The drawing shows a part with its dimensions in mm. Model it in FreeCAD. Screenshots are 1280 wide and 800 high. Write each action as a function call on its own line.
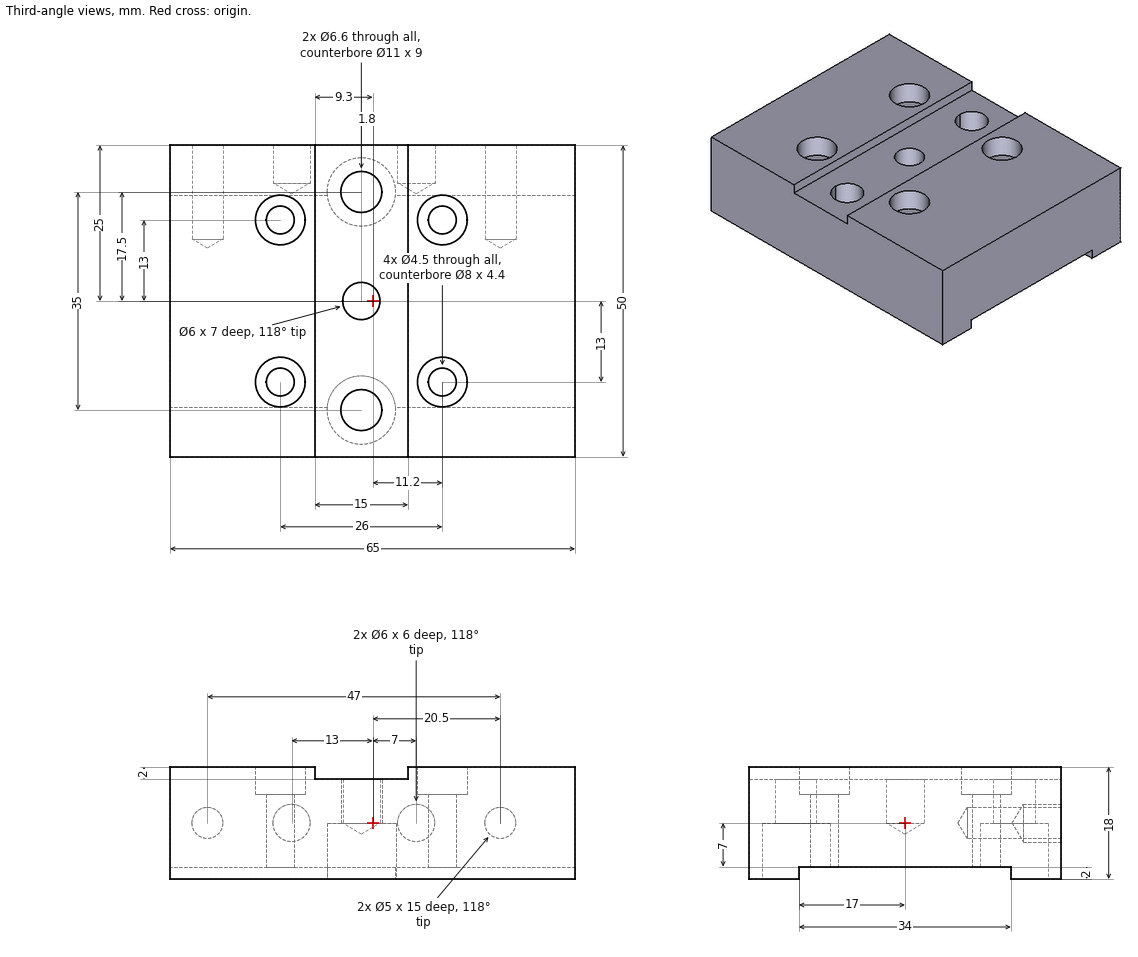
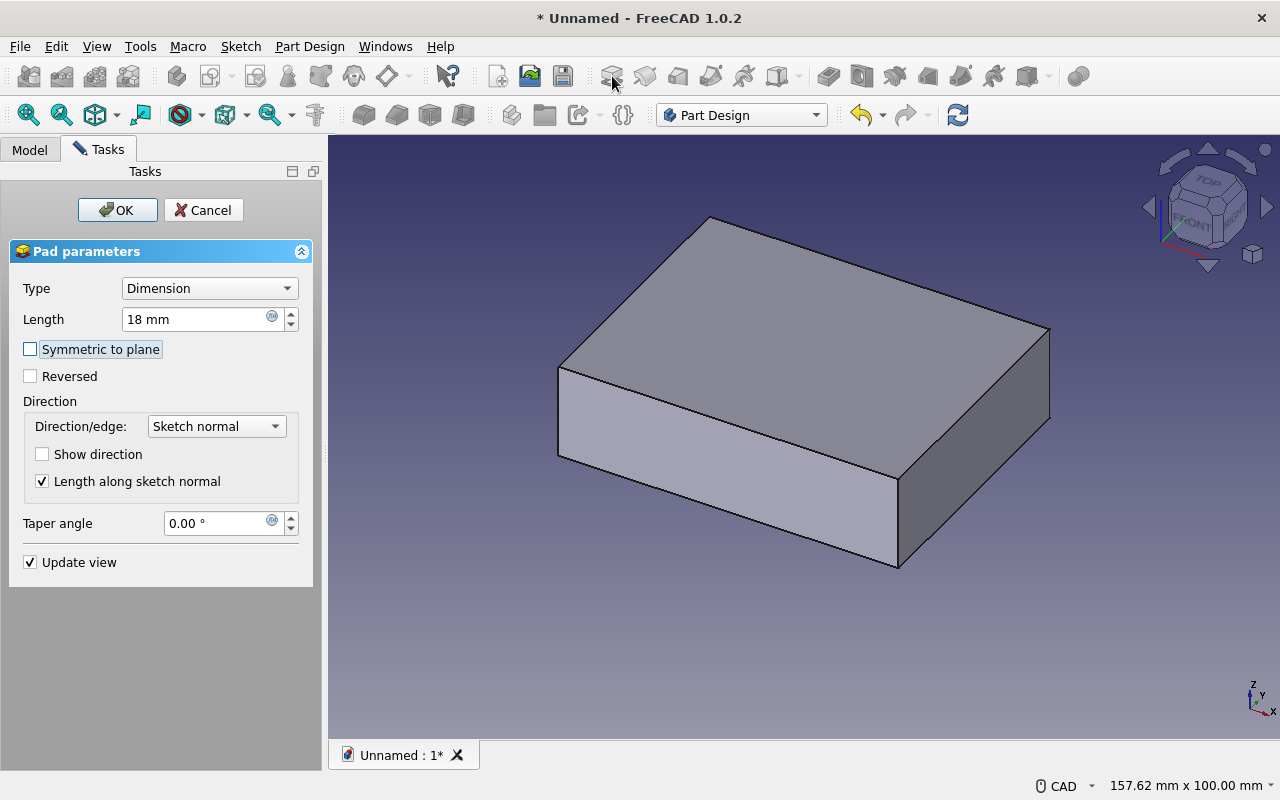
click(31, 349)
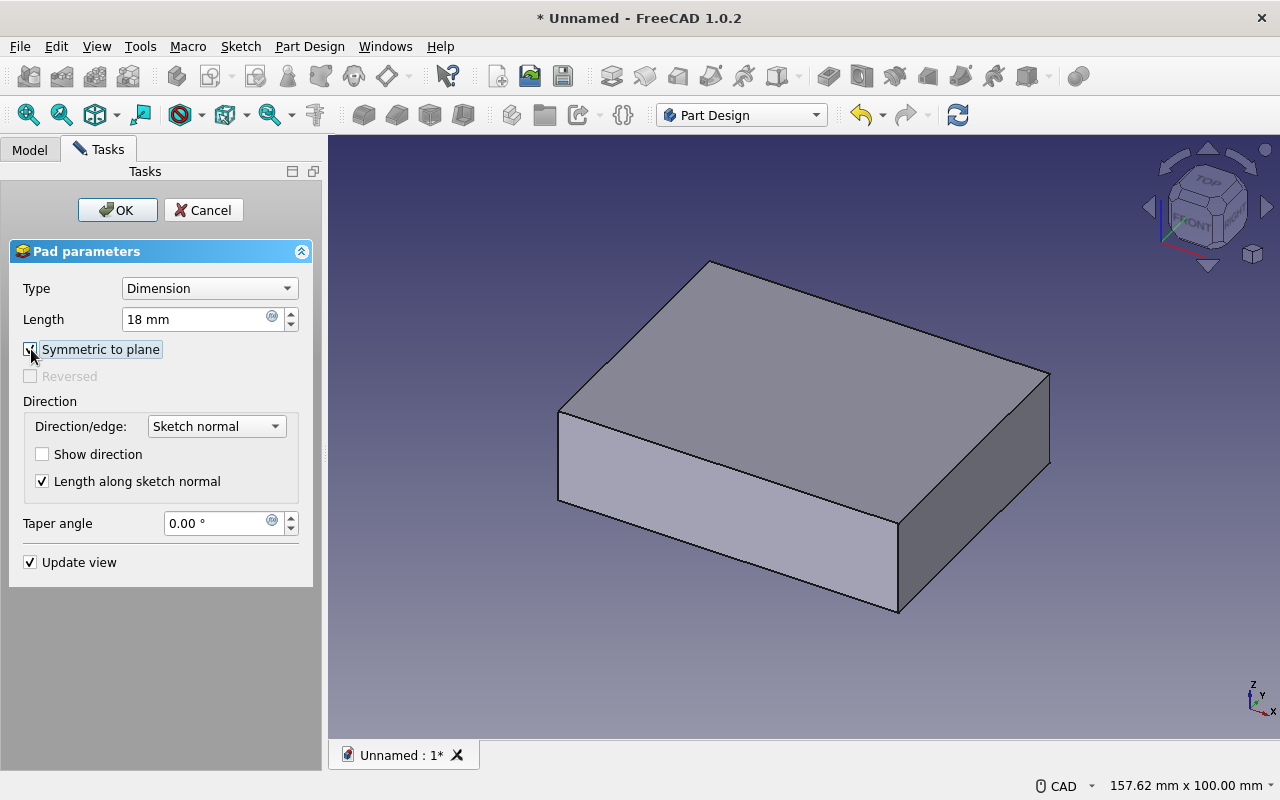
click(118, 210)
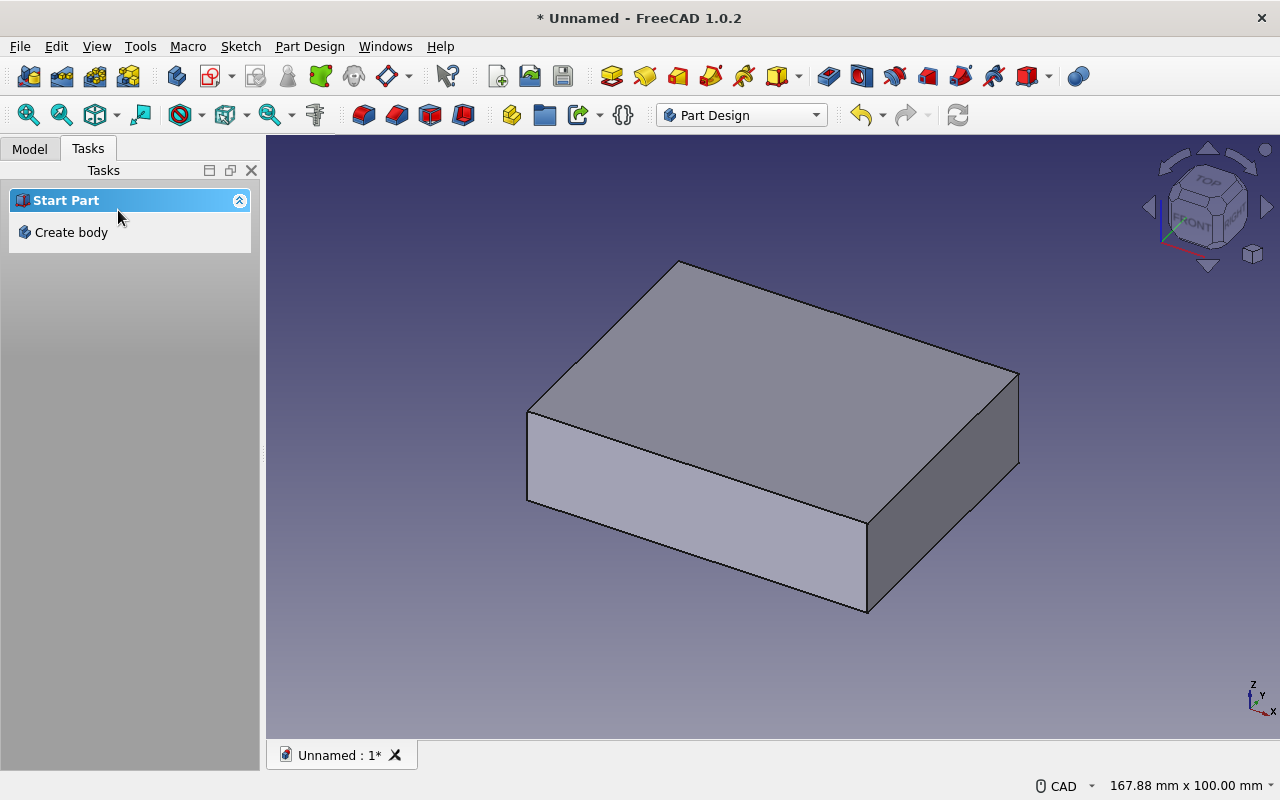
click(986, 449)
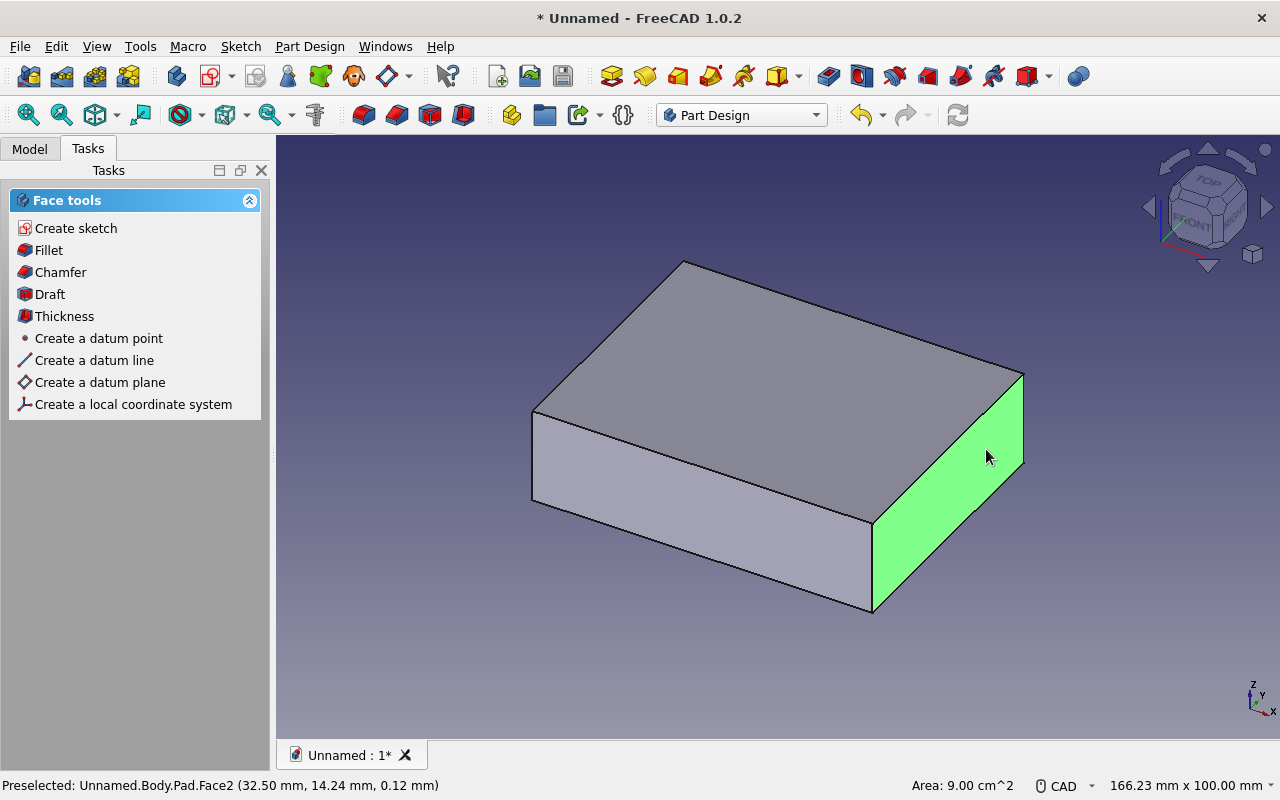
click(210, 76)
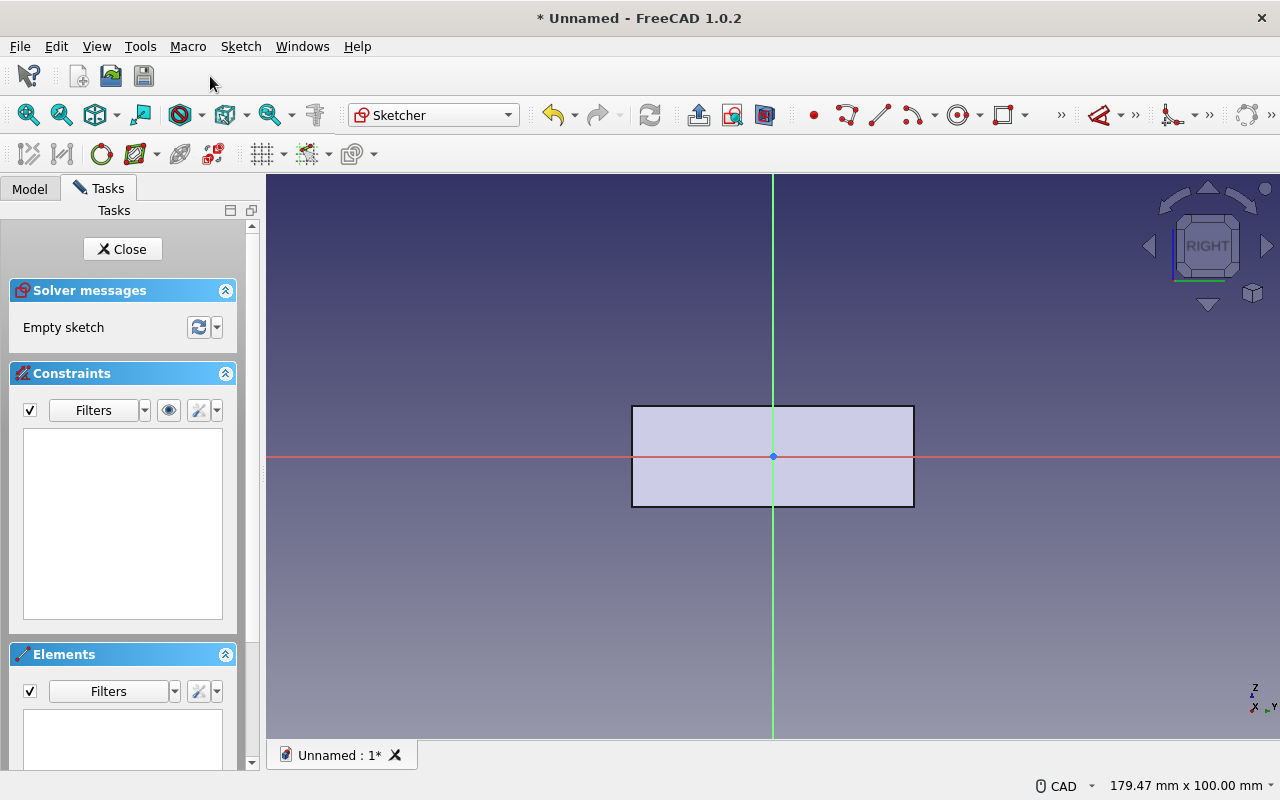
scroll(803, 493, up, 6)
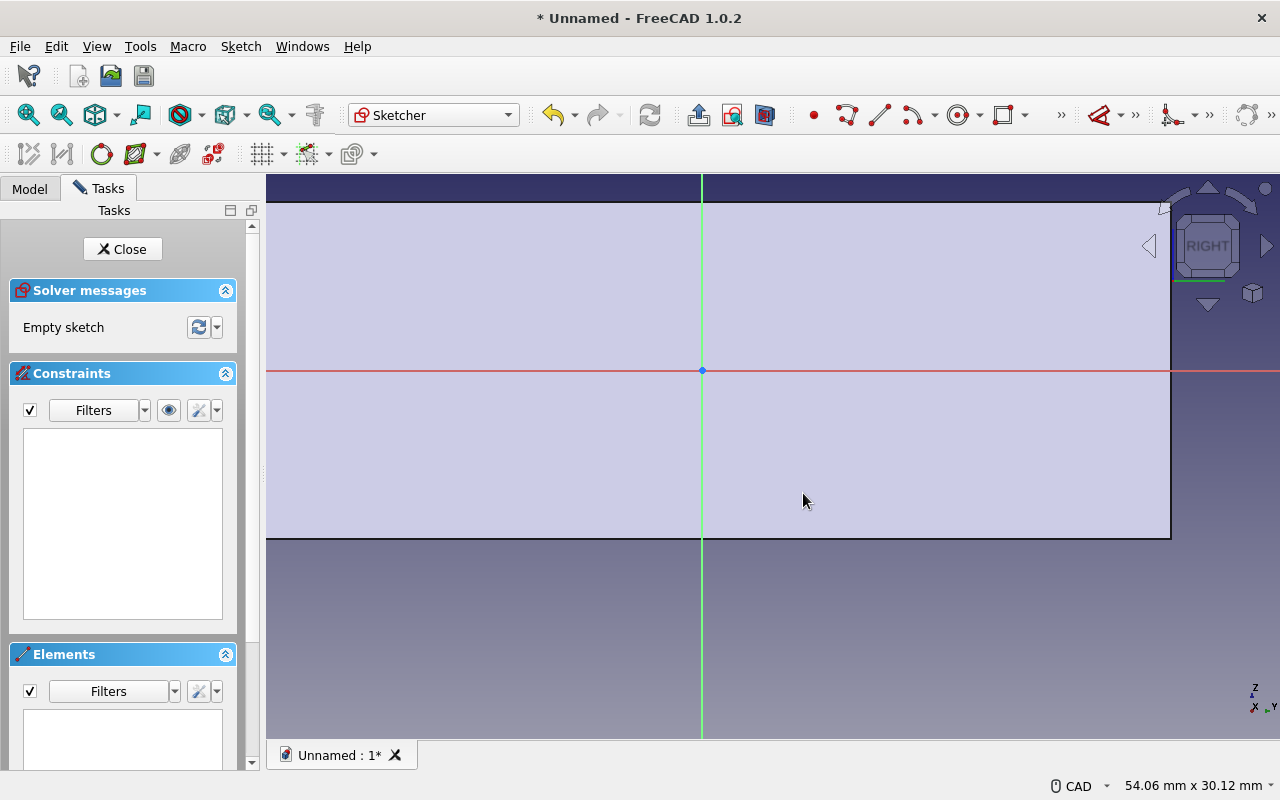
key(g)
key(r)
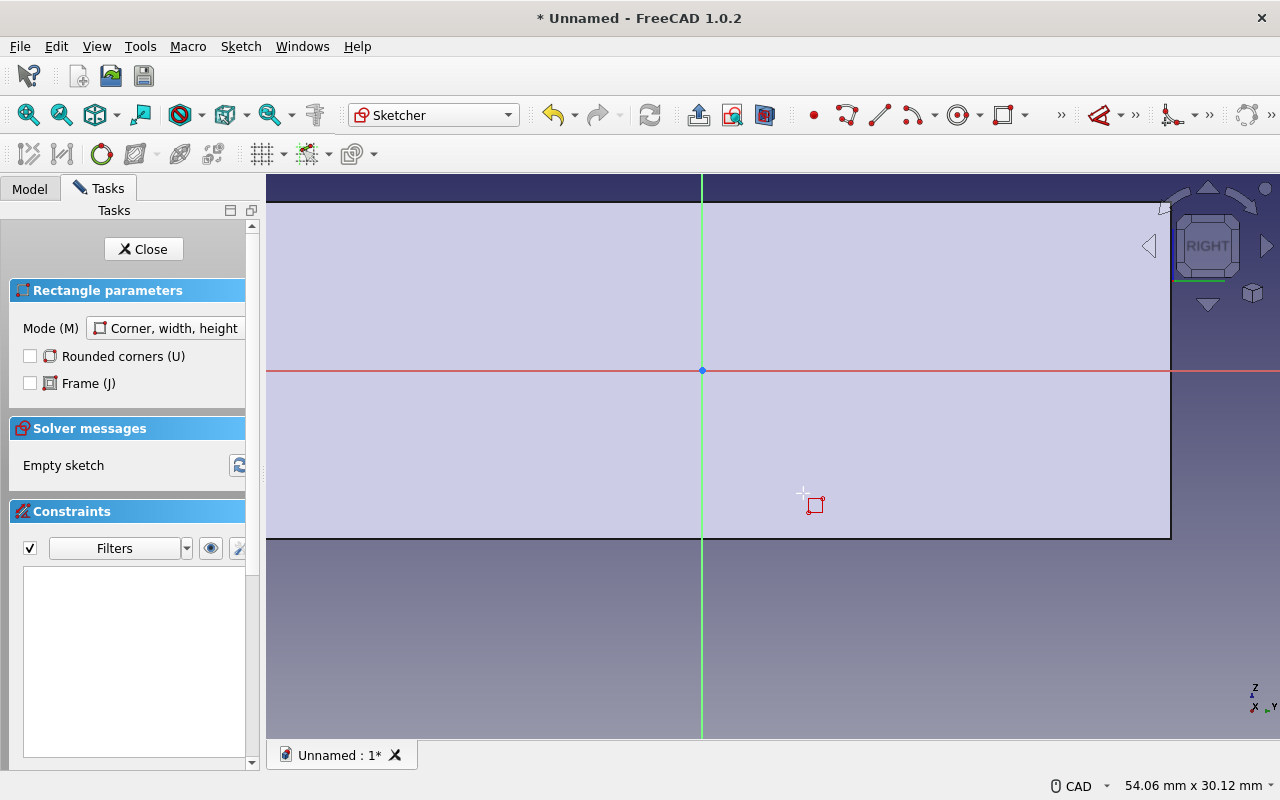
click(383, 502)
move(1021, 539)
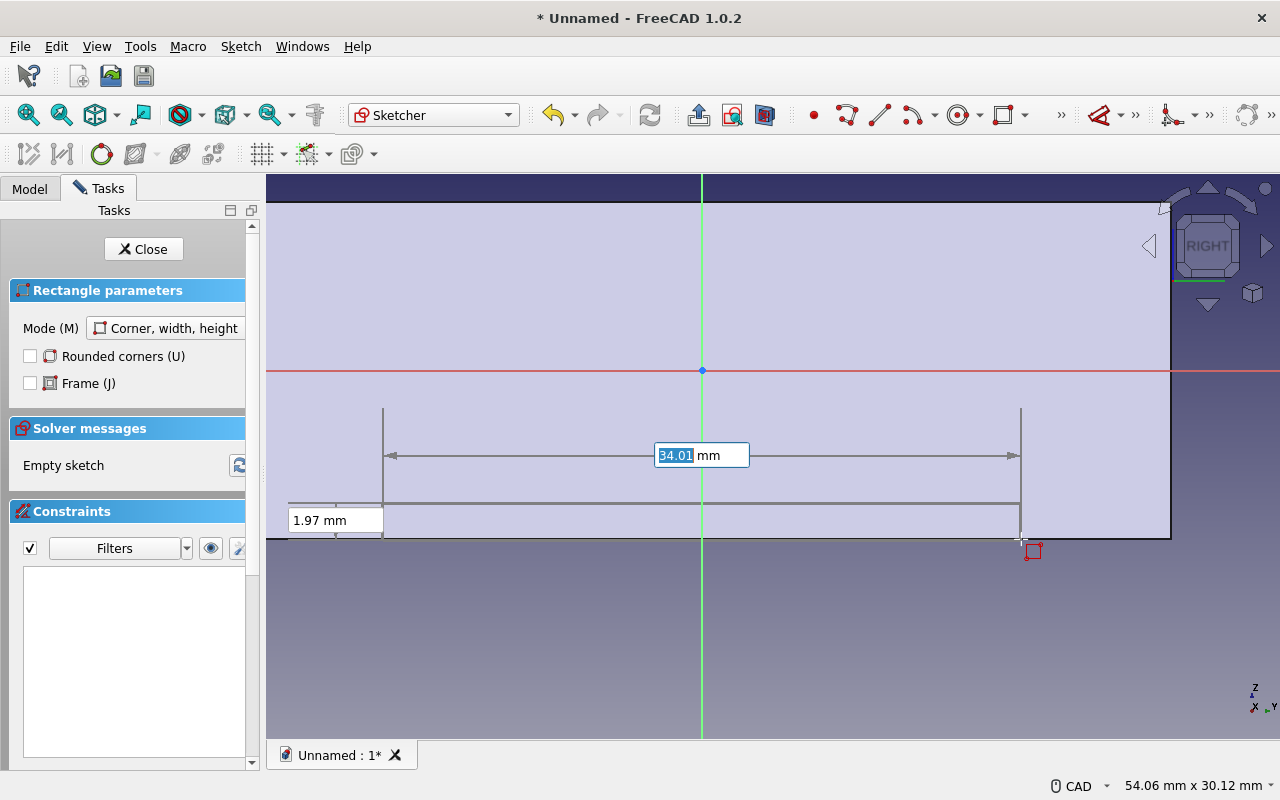
text(34)
key(Tab)
text(2)
key(Return)
key(Escape)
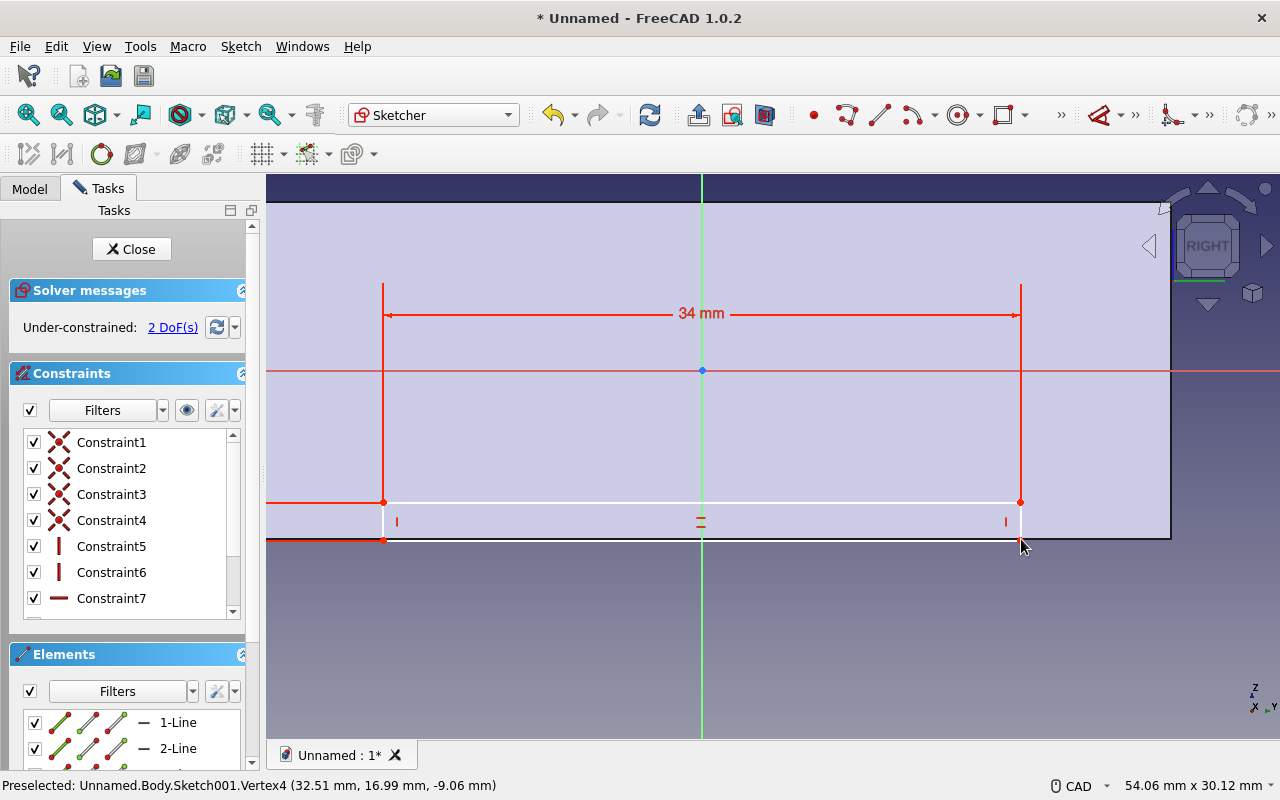
click(1098, 116)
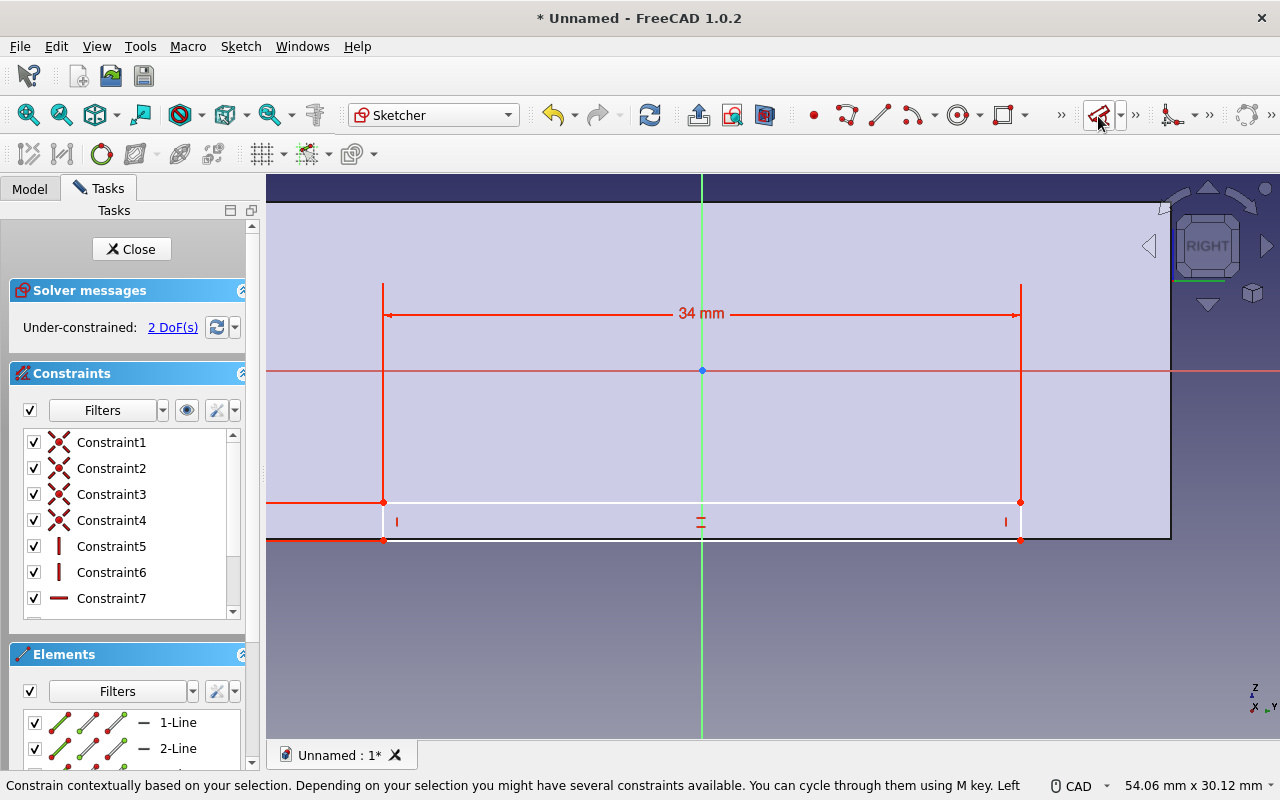
click(383, 503)
click(349, 437)